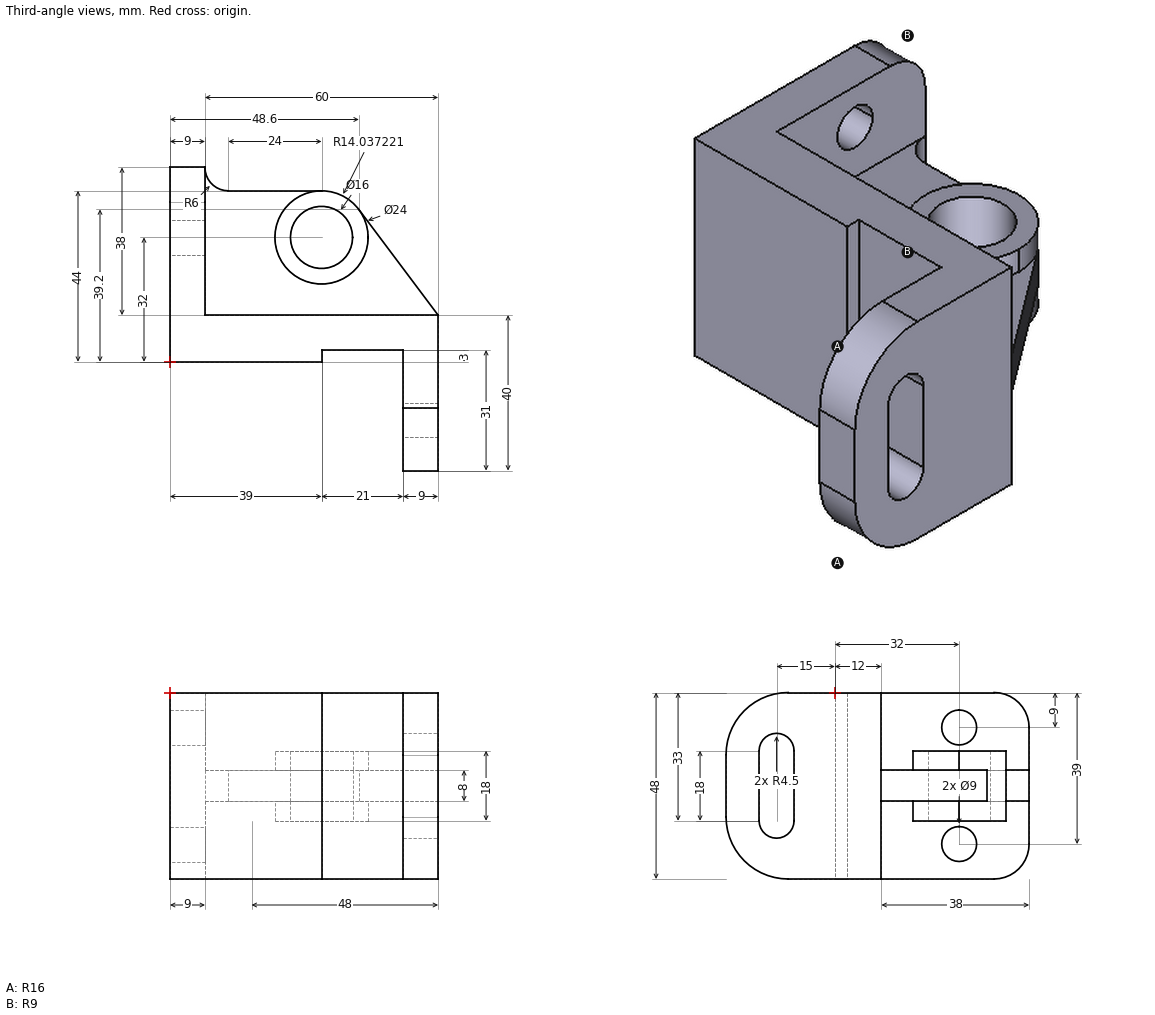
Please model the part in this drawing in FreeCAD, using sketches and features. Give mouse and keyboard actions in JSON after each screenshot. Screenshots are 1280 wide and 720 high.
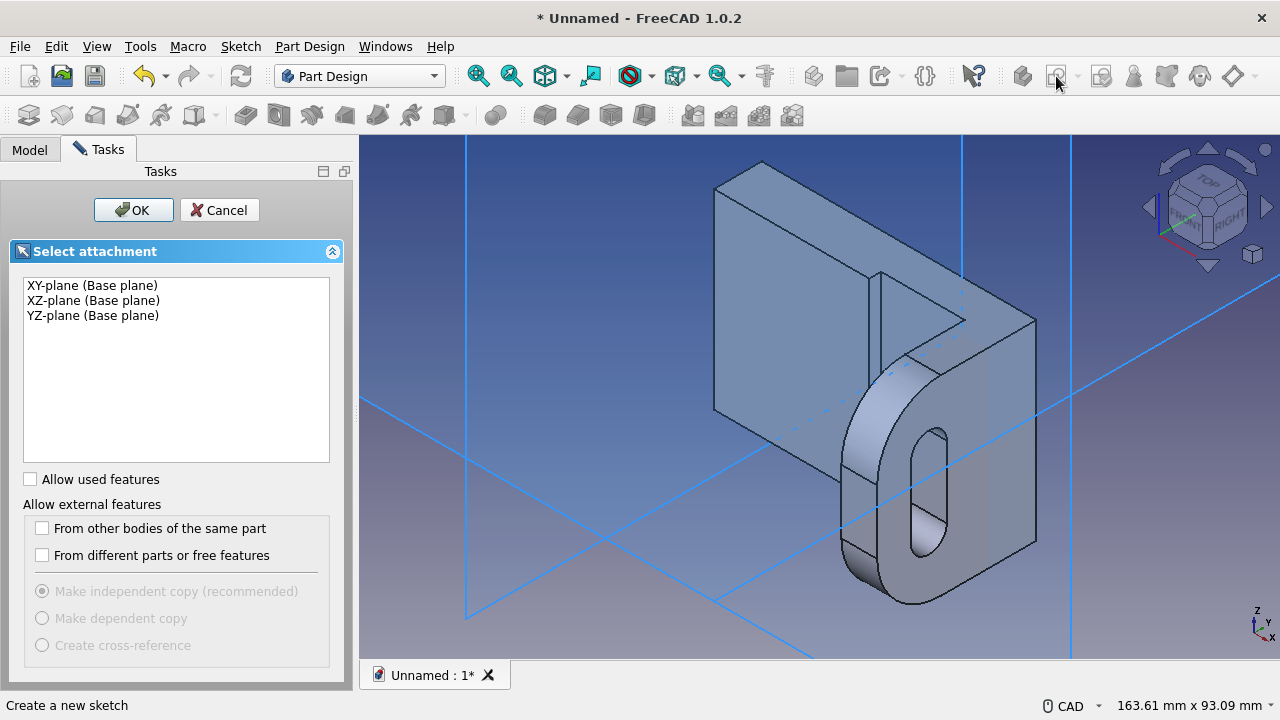
{"action": "left_click", "coordinate": [84, 316]}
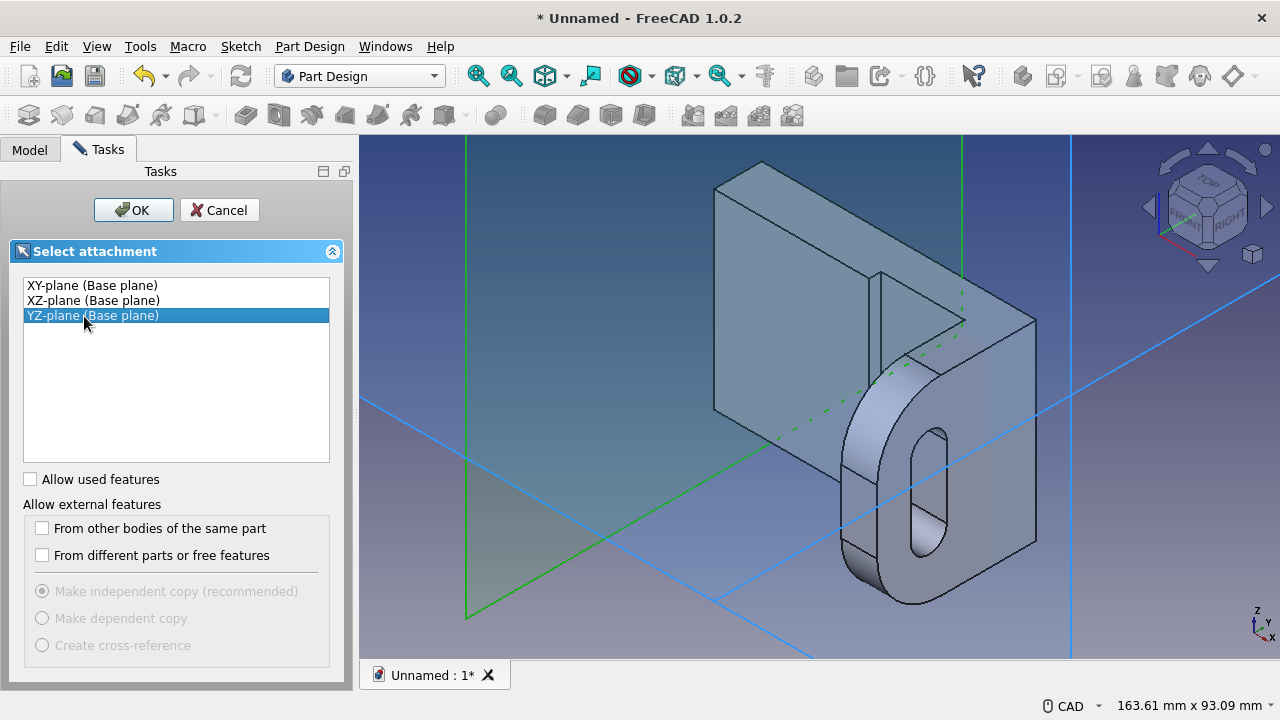
{"action": "left_click", "coordinate": [134, 210]}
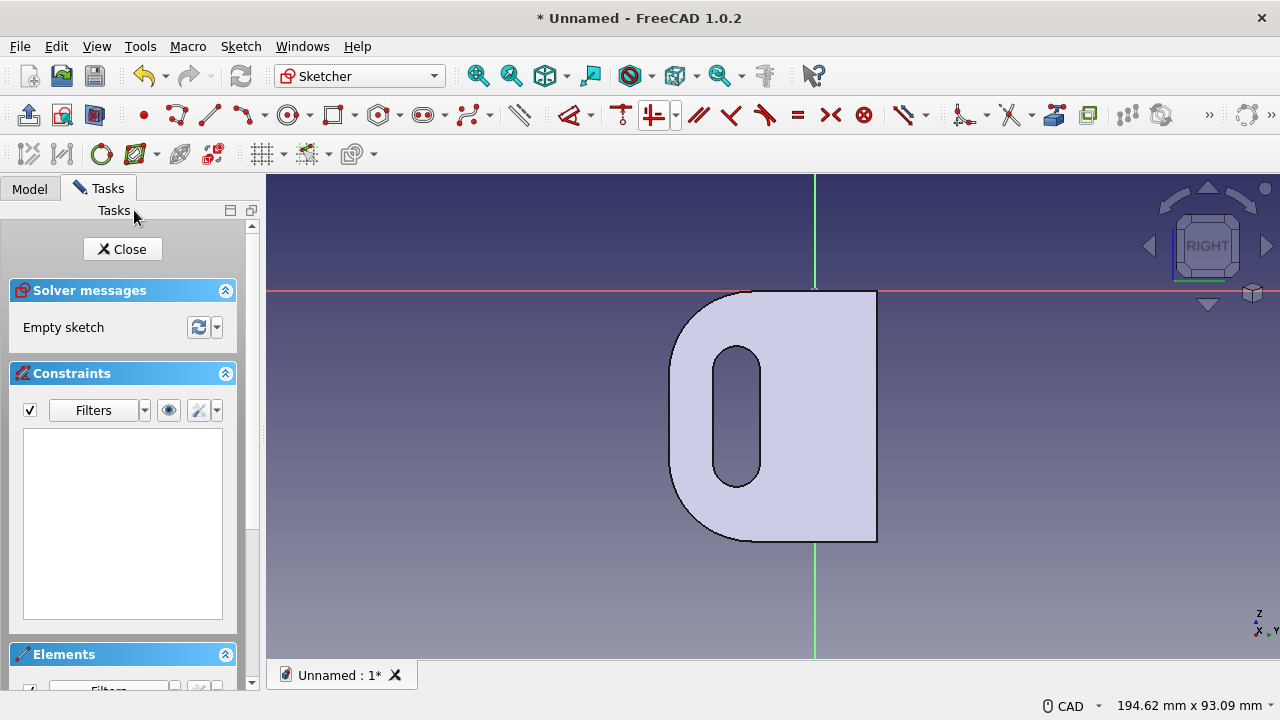
{"action": "key", "text": "q s"}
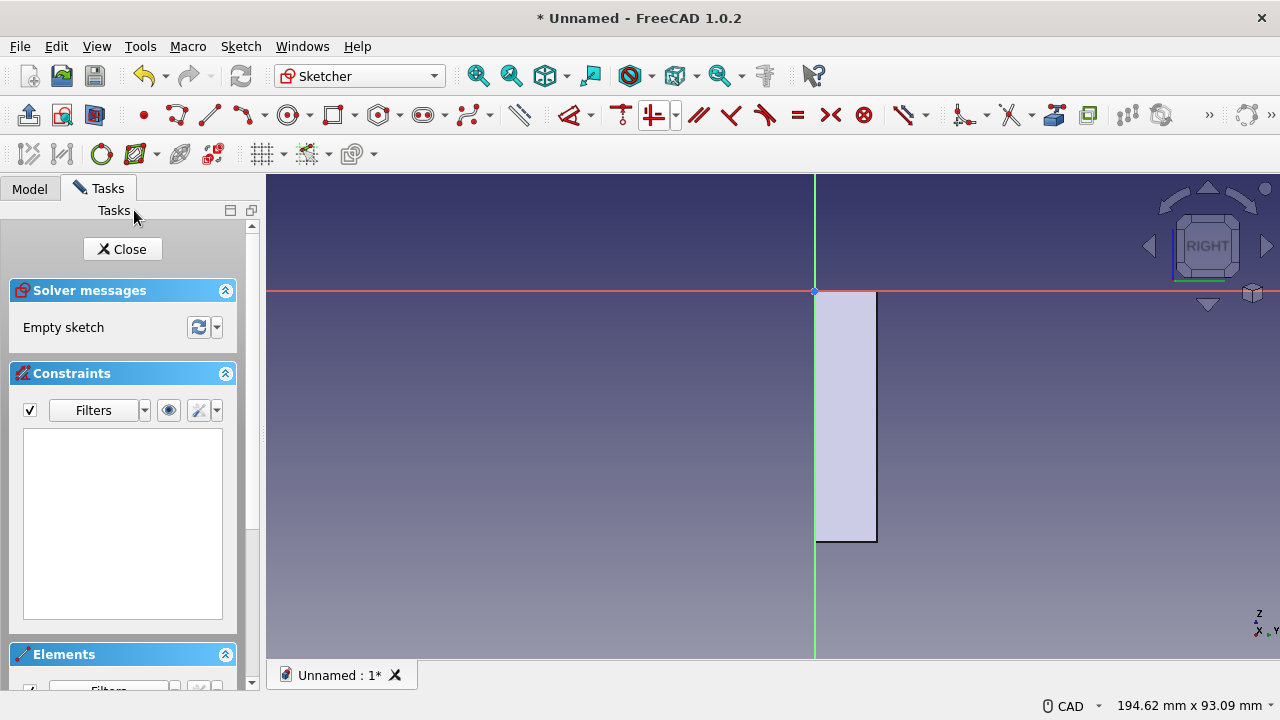
{"action": "key", "text": "g r"}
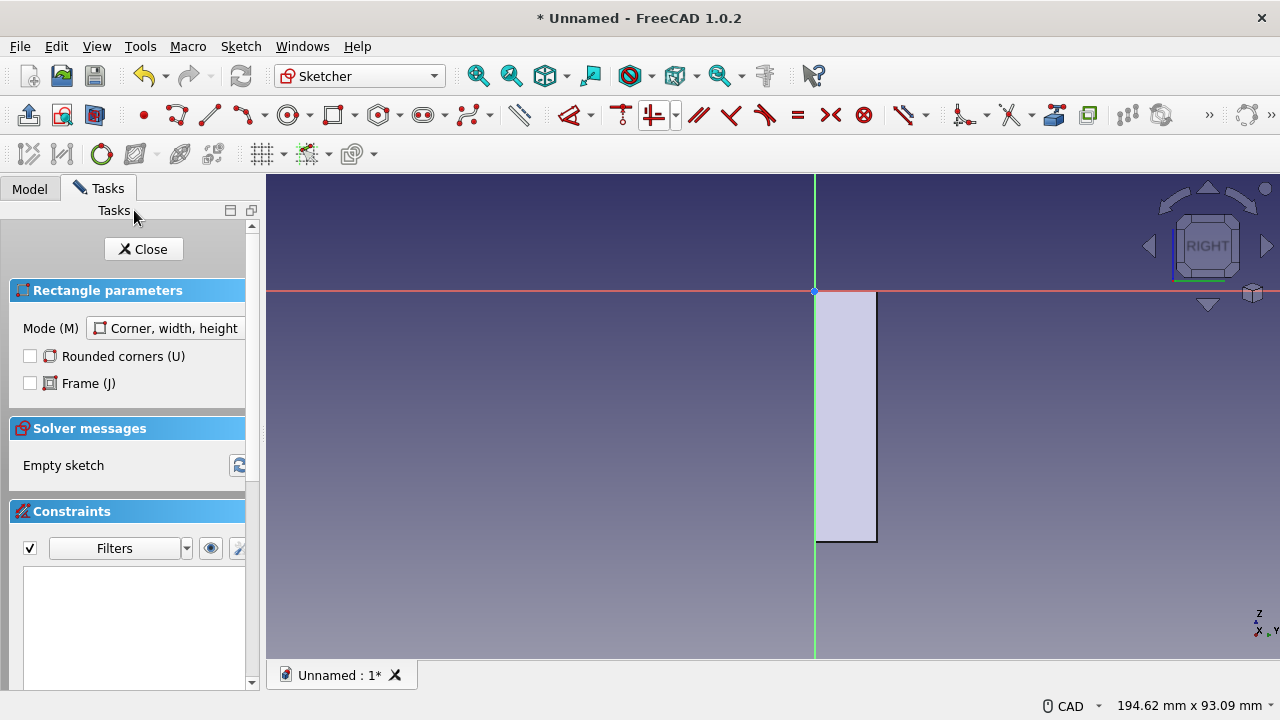
{"action": "left_click", "coordinate": [877, 291]}
{"action": "left_click", "coordinate": [1075, 542]}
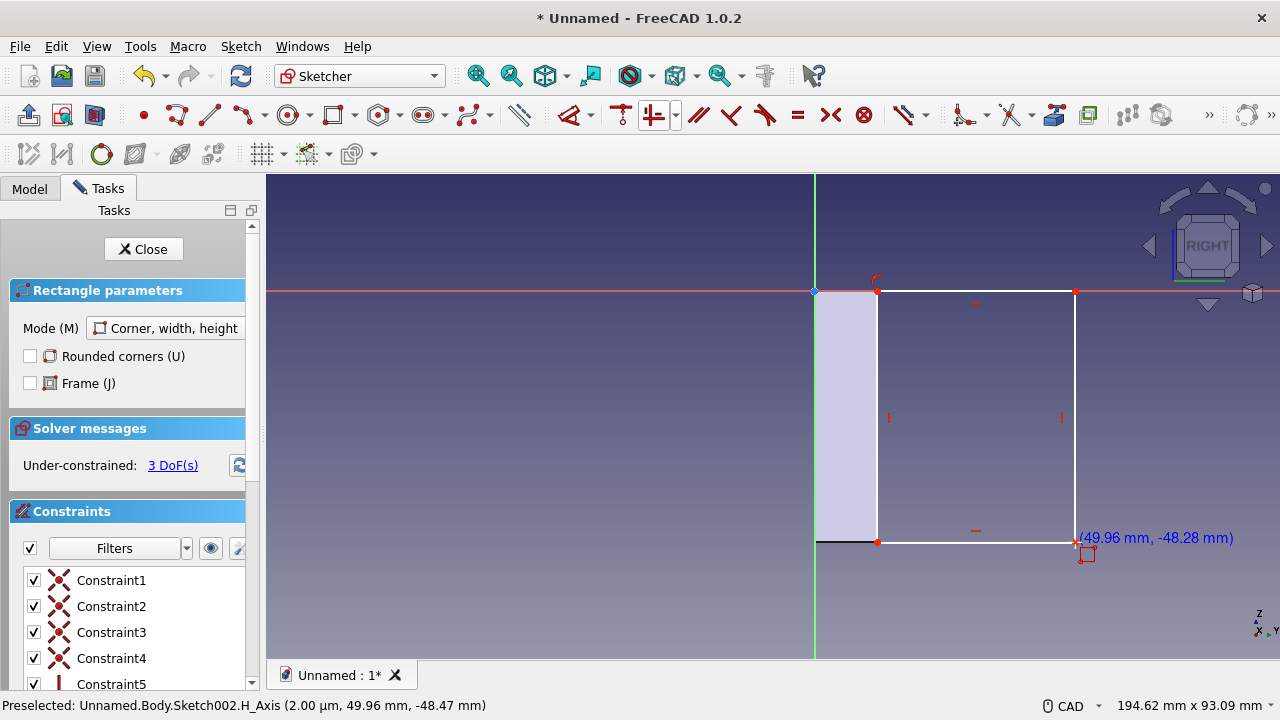
{"action": "key", "text": "g c"}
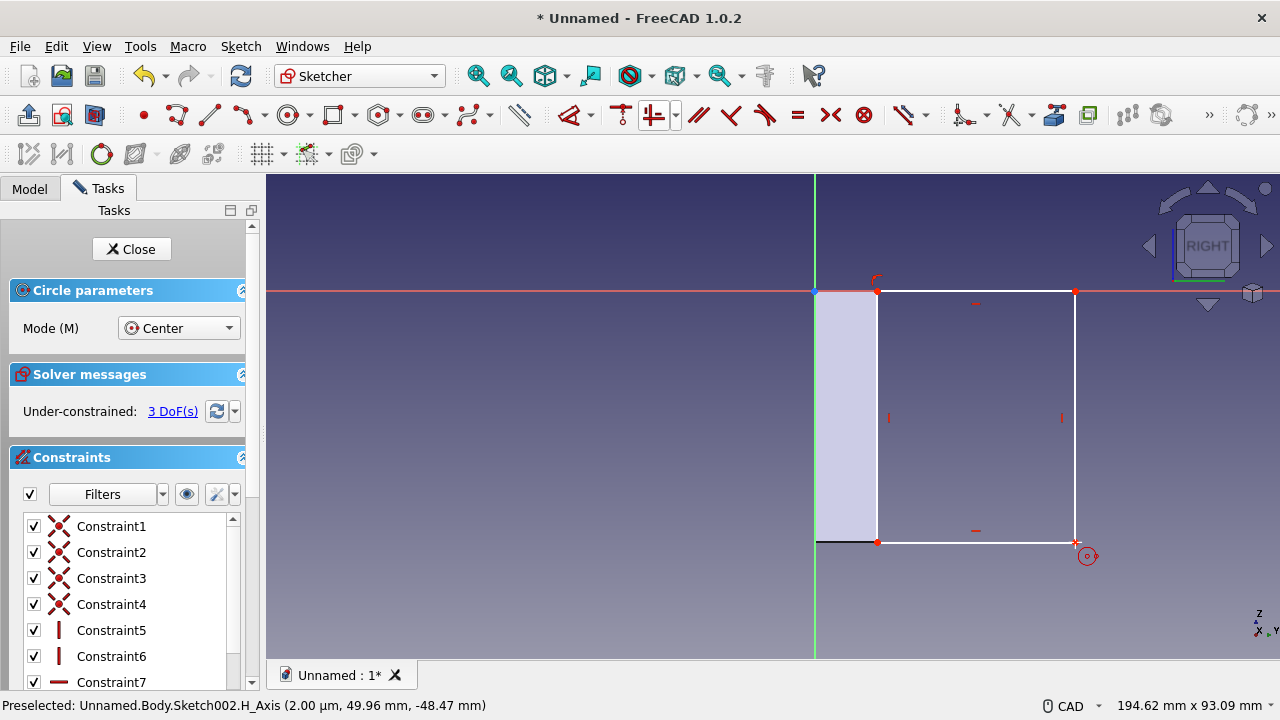
{"action": "left_click", "coordinate": [981, 495]}
{"action": "left_click", "coordinate": [998, 478]}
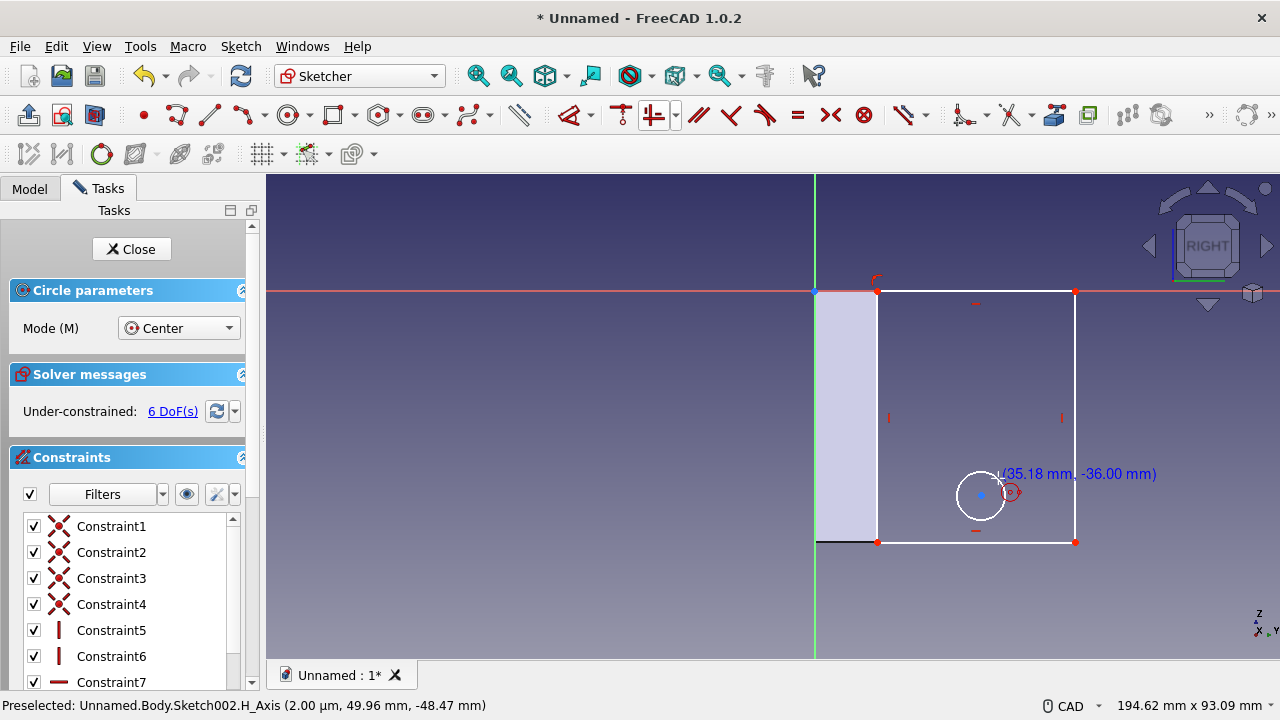
{"action": "left_click", "coordinate": [981, 338]}
{"action": "left_click", "coordinate": [998, 322]}
{"action": "key", "text": "Escape"}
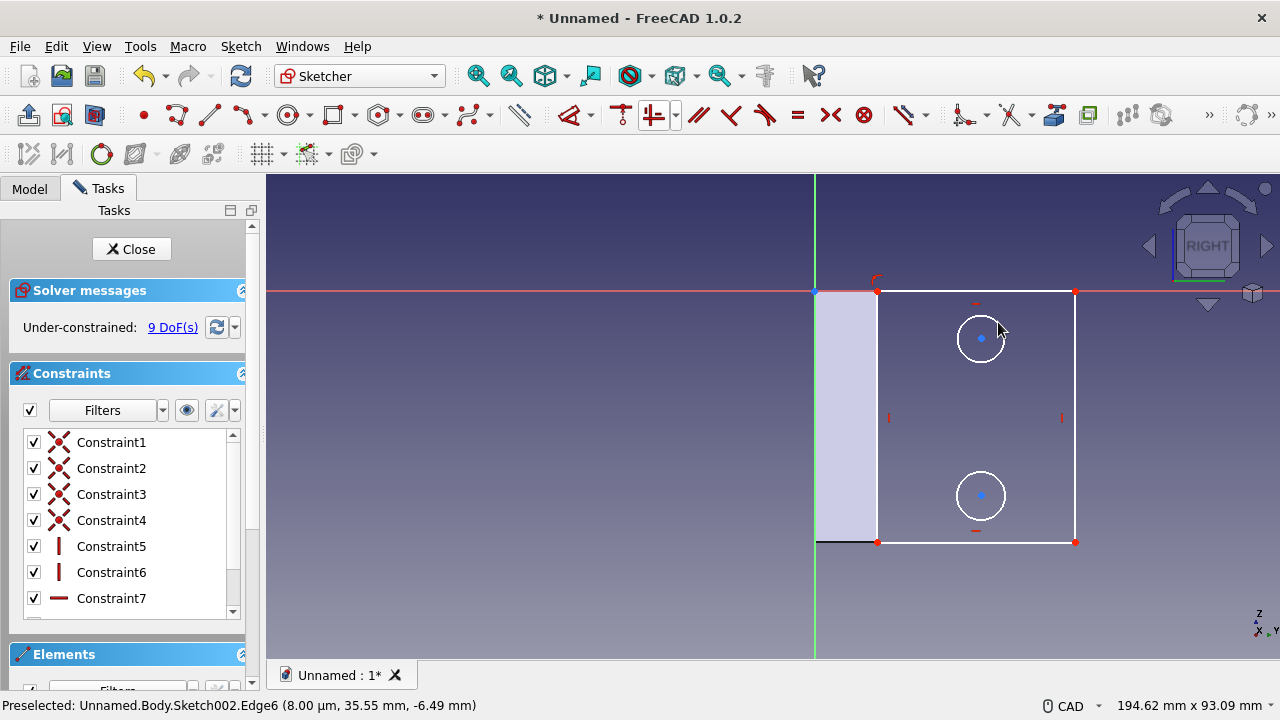
{"action": "left_click", "coordinate": [998, 479]}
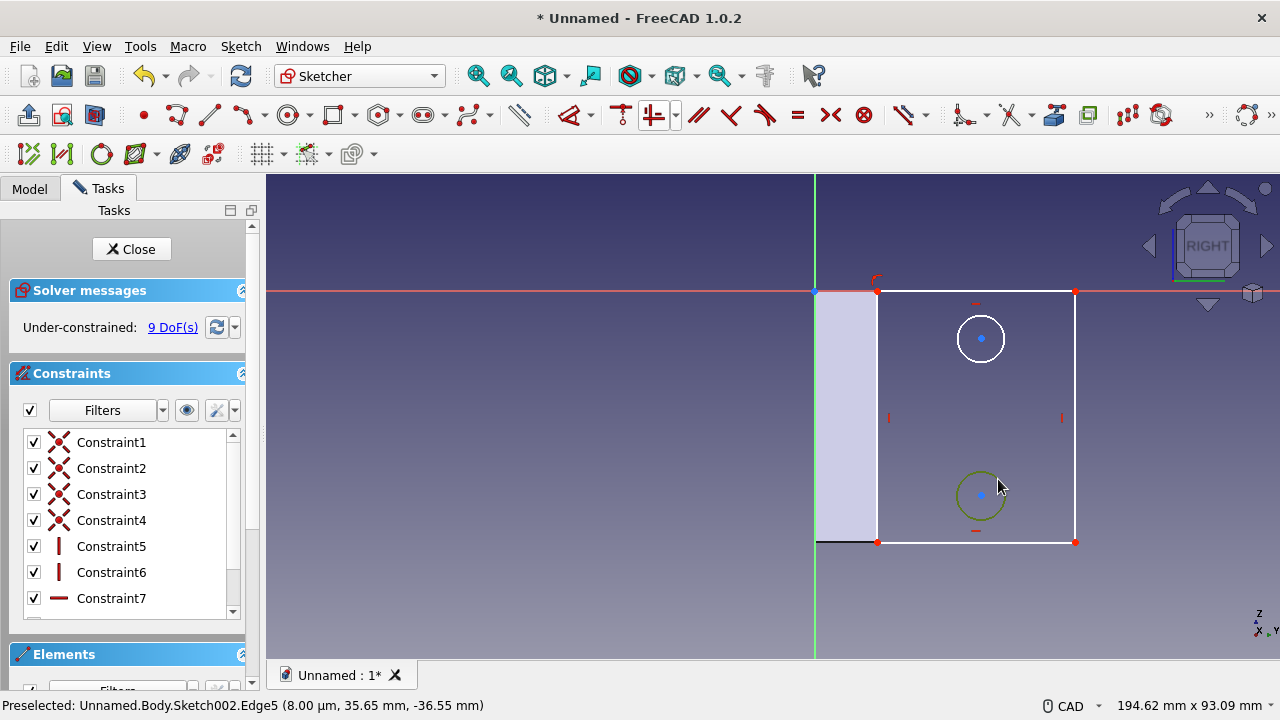
{"action": "left_click", "coordinate": [997, 322]}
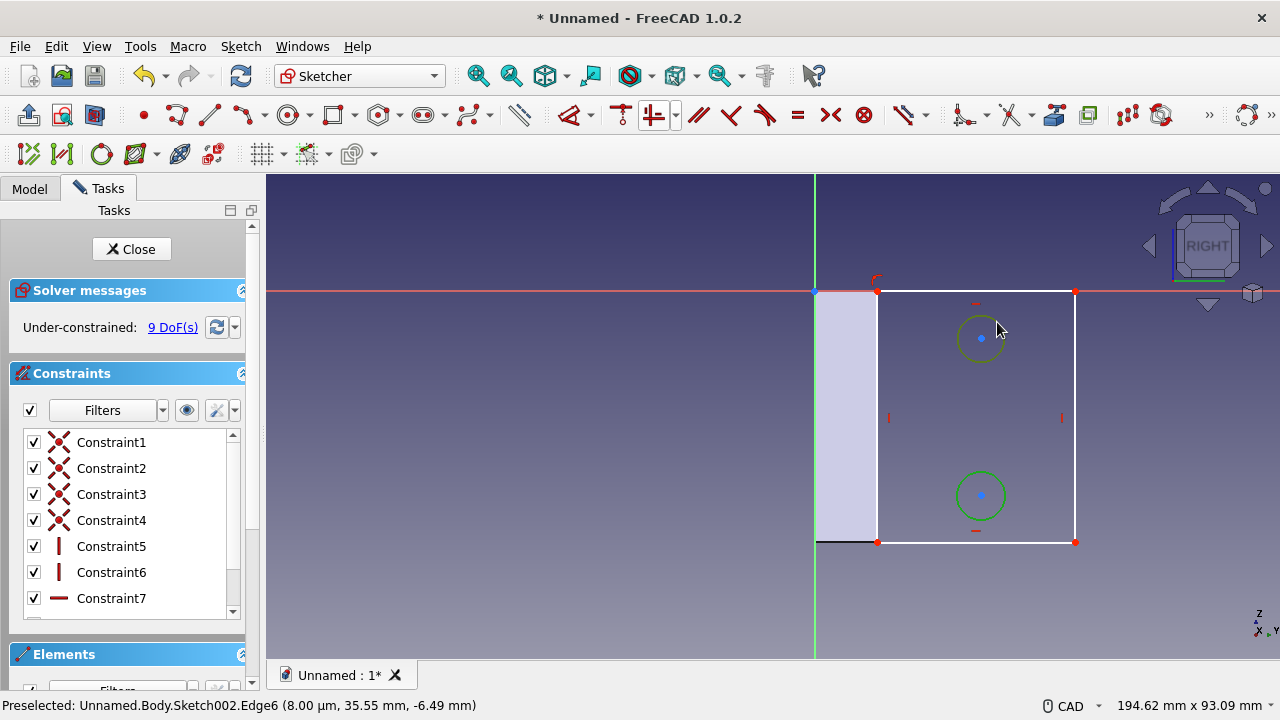
{"action": "left_click", "coordinate": [798, 116]}